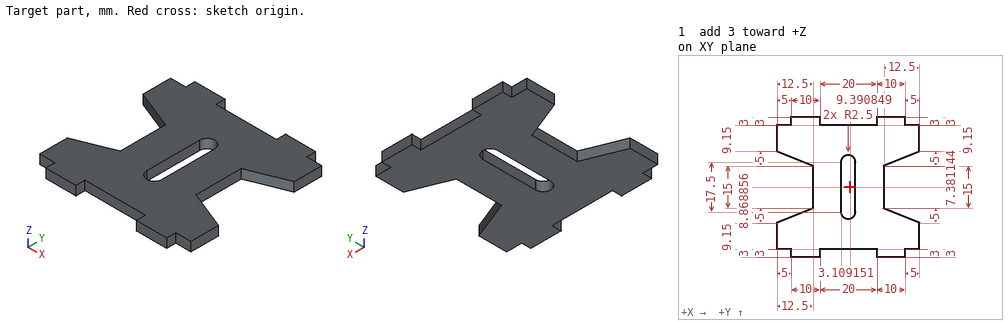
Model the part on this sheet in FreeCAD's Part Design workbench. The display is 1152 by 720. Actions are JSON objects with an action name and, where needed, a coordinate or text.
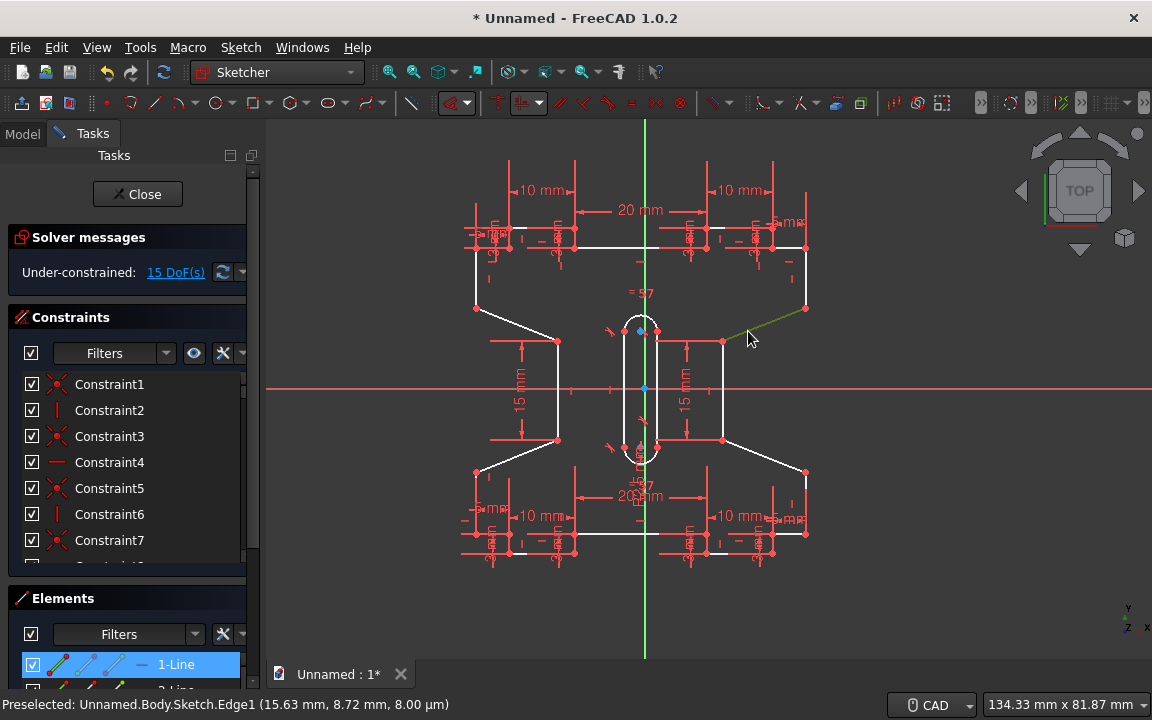
{"action": "left_click", "coordinate": [470, 104]}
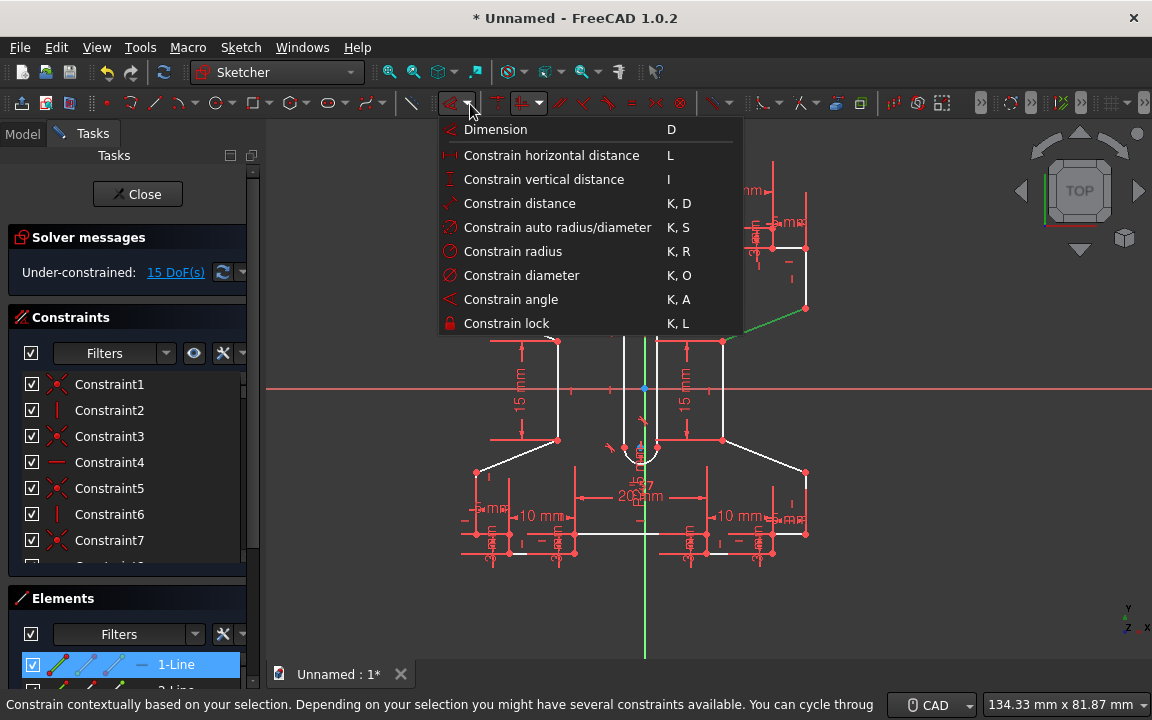
{"action": "left_click", "coordinate": [591, 179]}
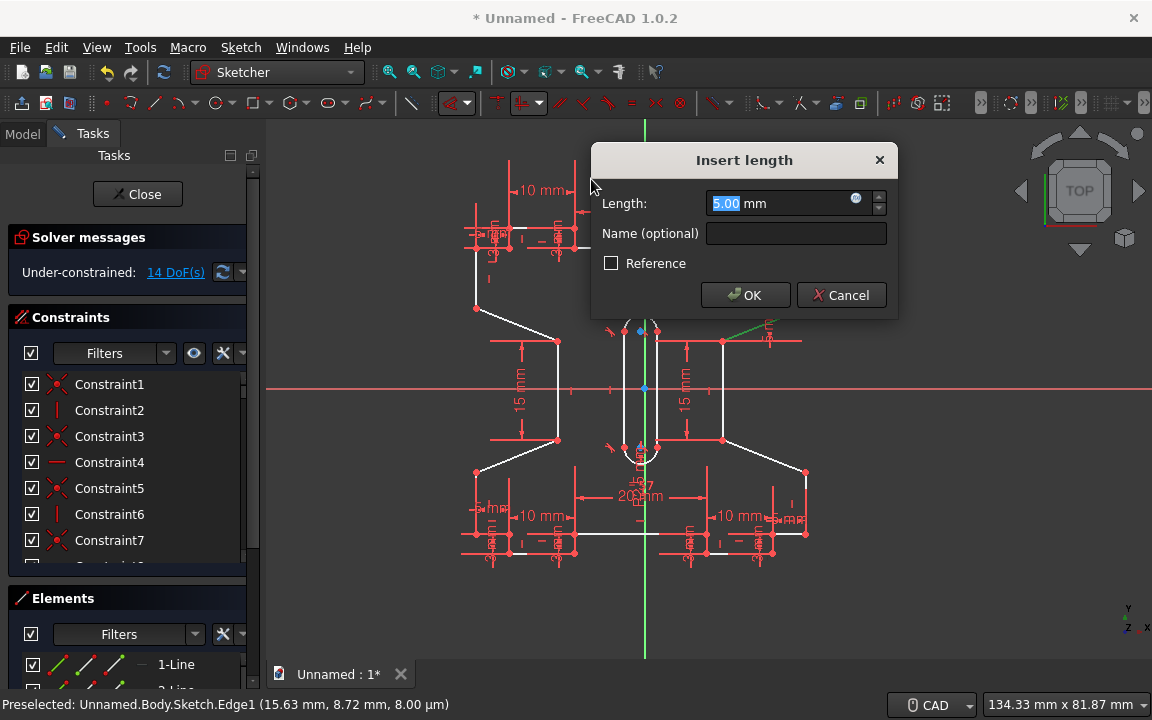
{"action": "type", "text": "5"}
{"action": "key", "text": "Return"}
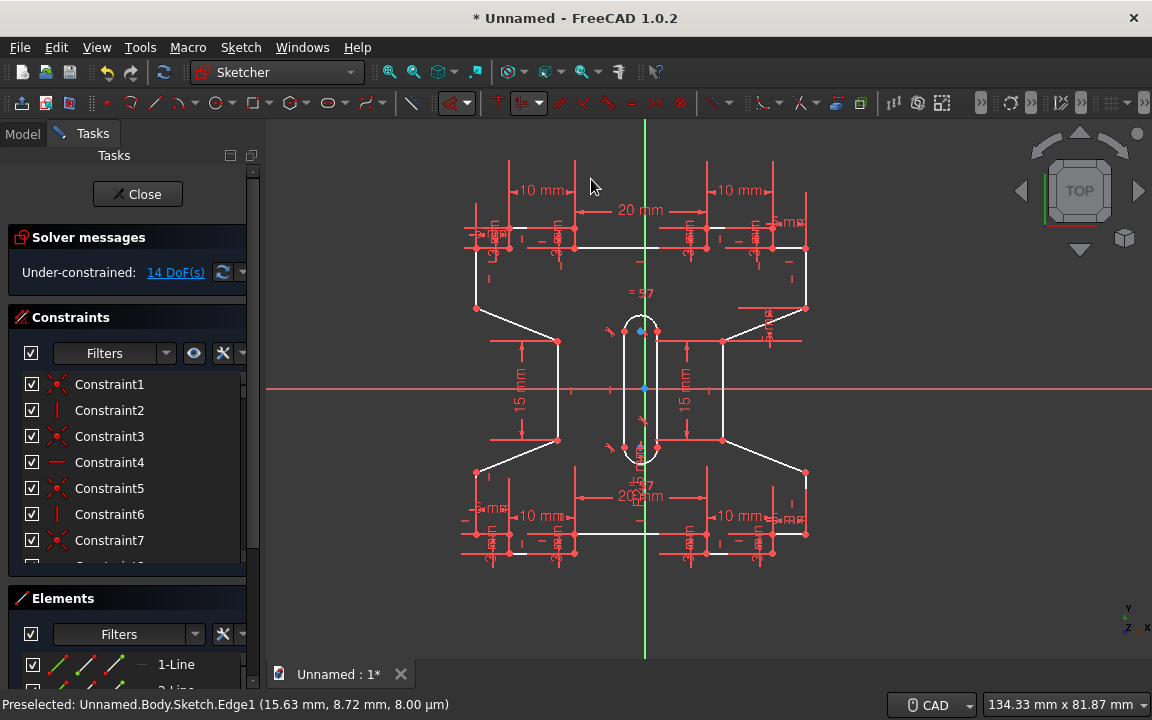
{"action": "left_click", "coordinate": [501, 318]}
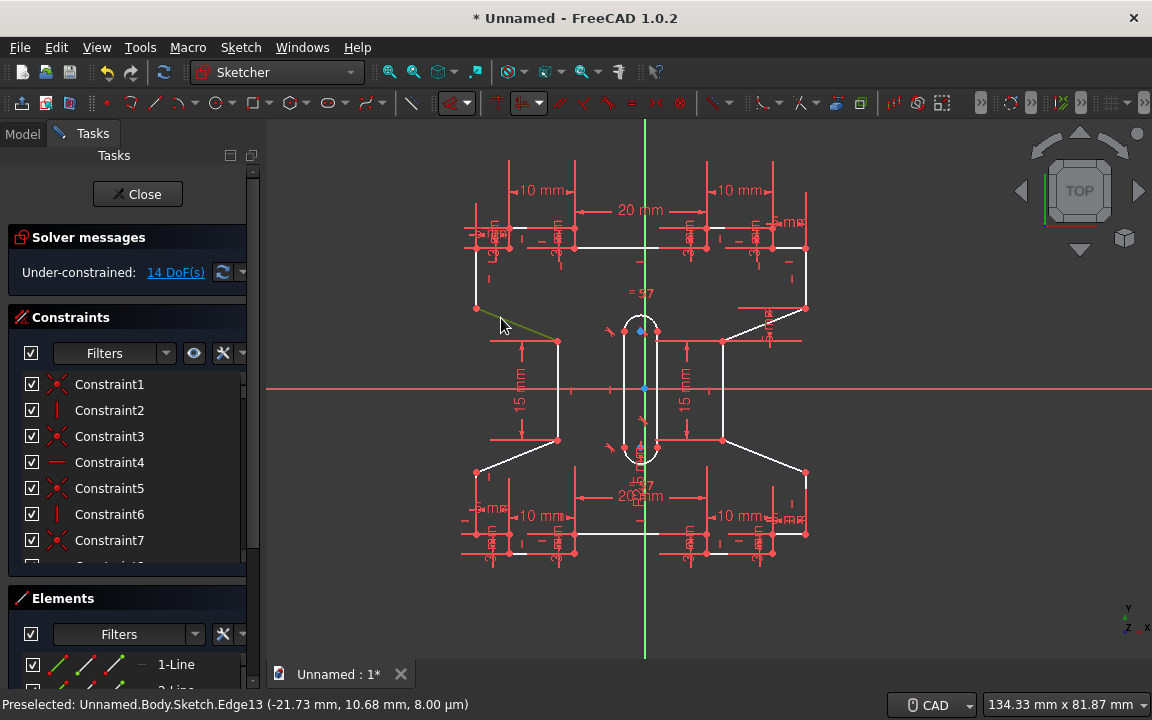
{"action": "left_click", "coordinate": [470, 104]}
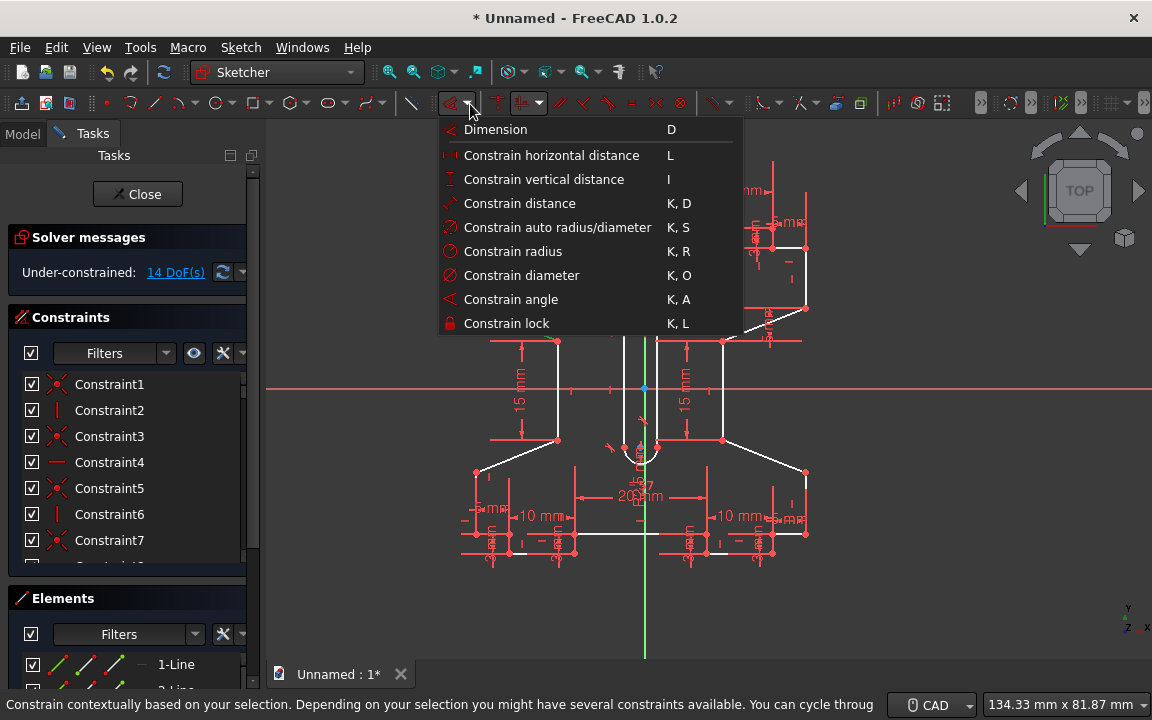
{"action": "left_click", "coordinate": [591, 179]}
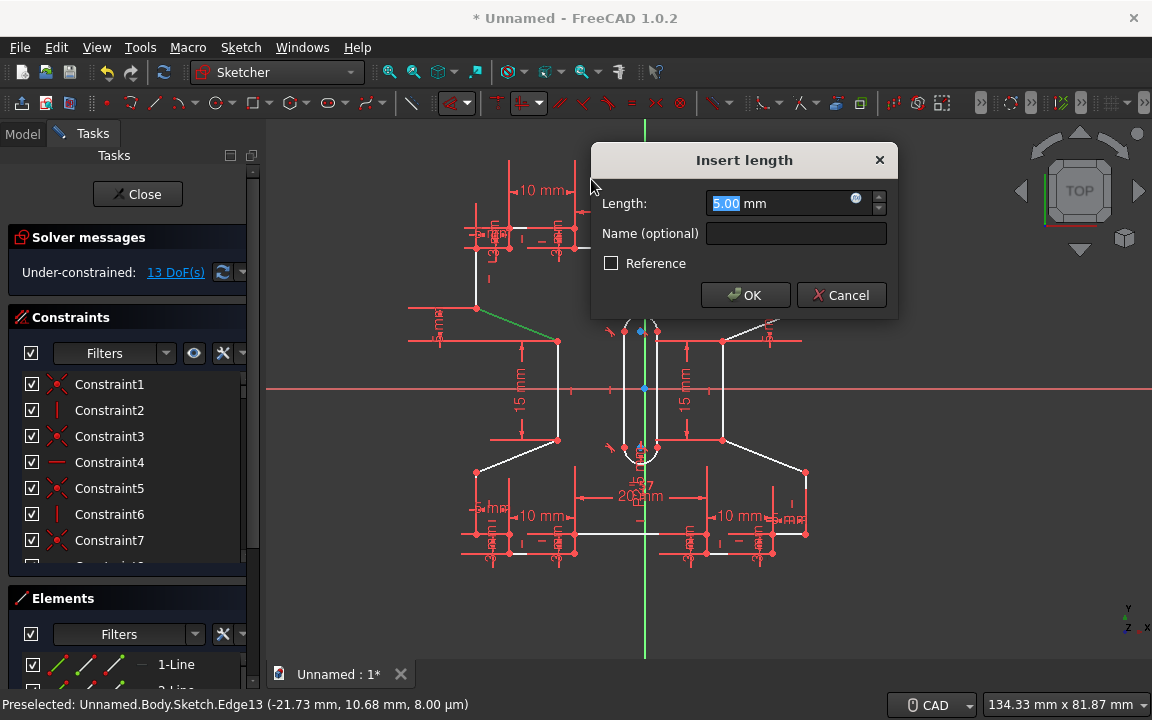
{"action": "type", "text": "5"}
{"action": "key", "text": "Return"}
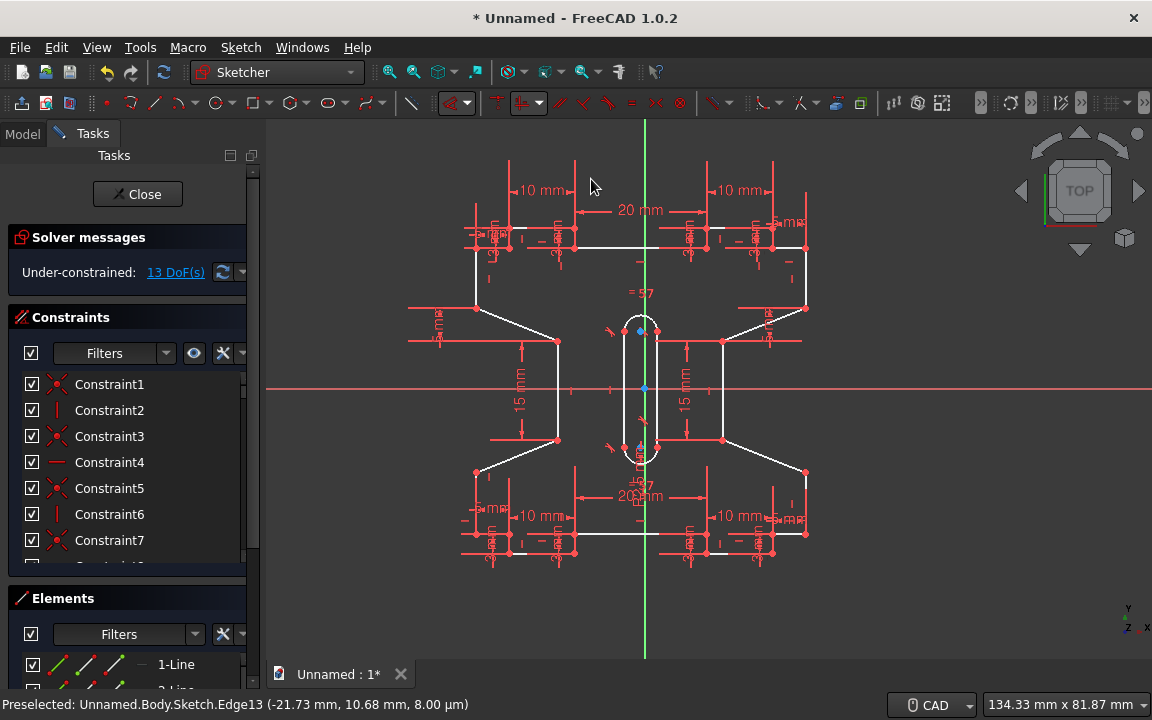
{"action": "left_click", "coordinate": [533, 450]}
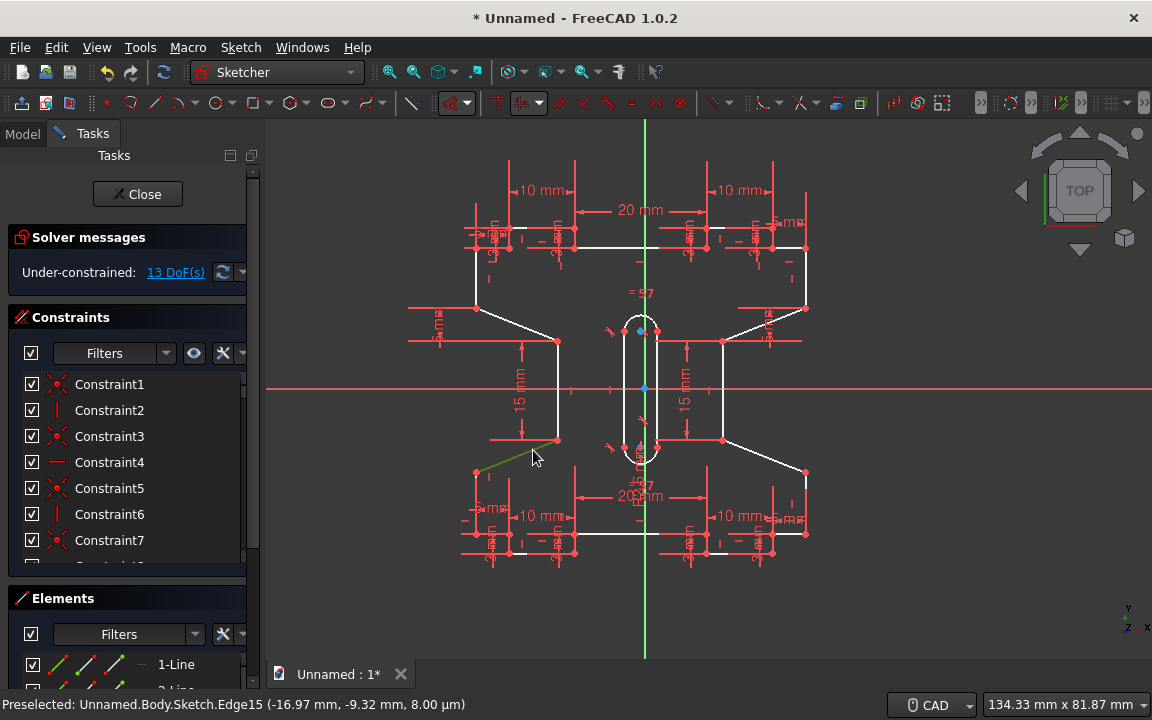
{"action": "key", "text": "i"}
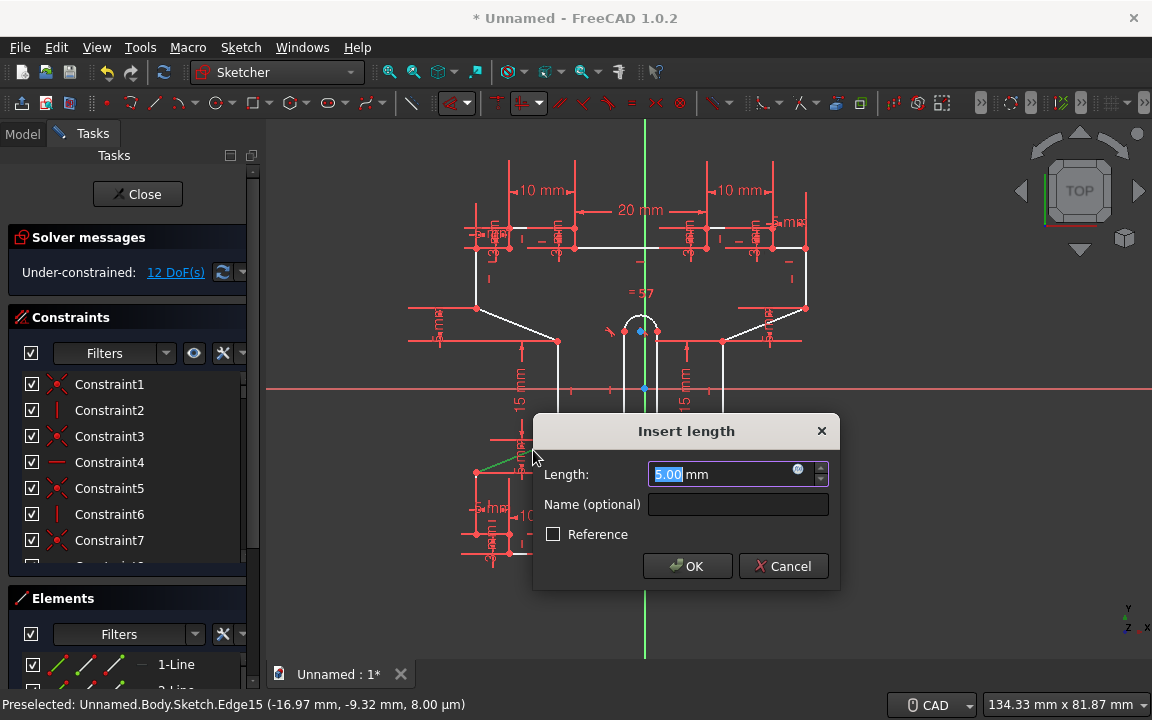
{"action": "type", "text": "5"}
{"action": "key", "text": "Return"}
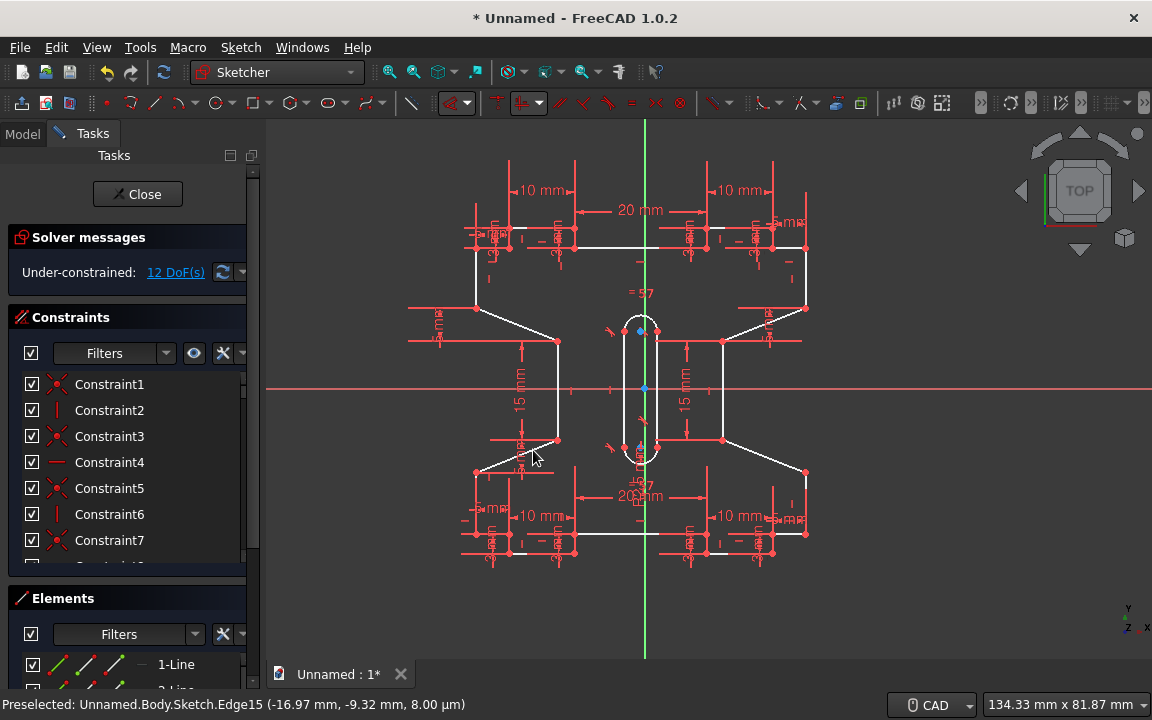
{"action": "left_click", "coordinate": [781, 463]}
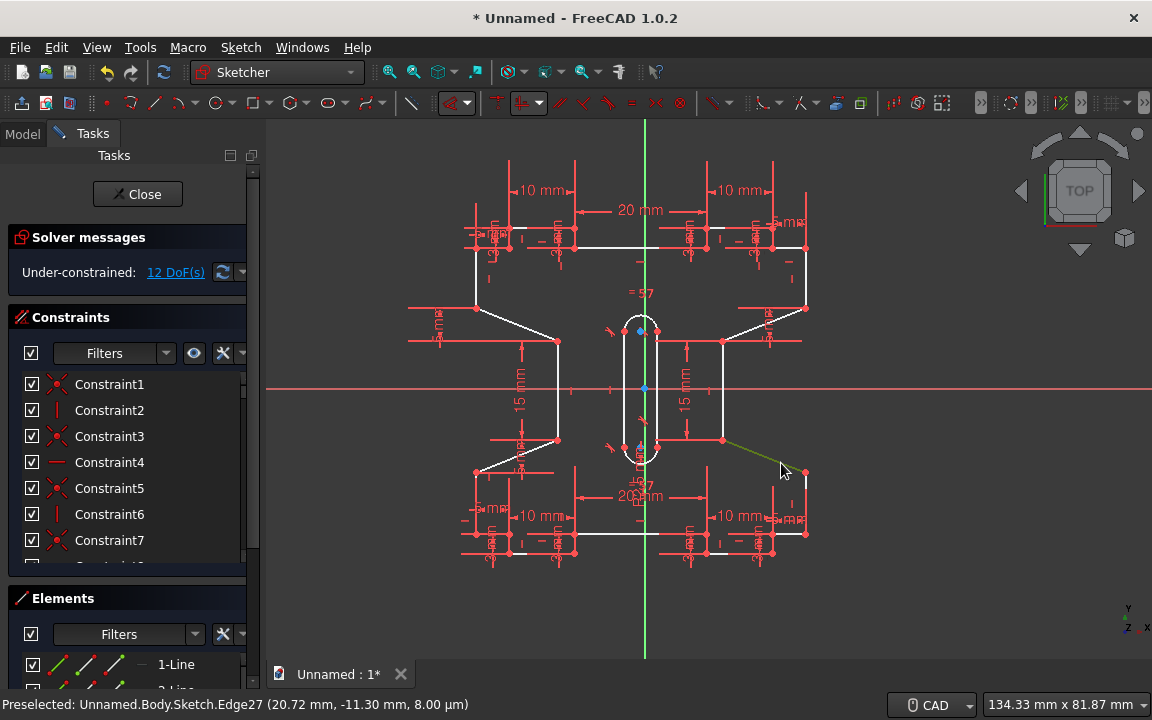
{"action": "left_click", "coordinate": [470, 104]}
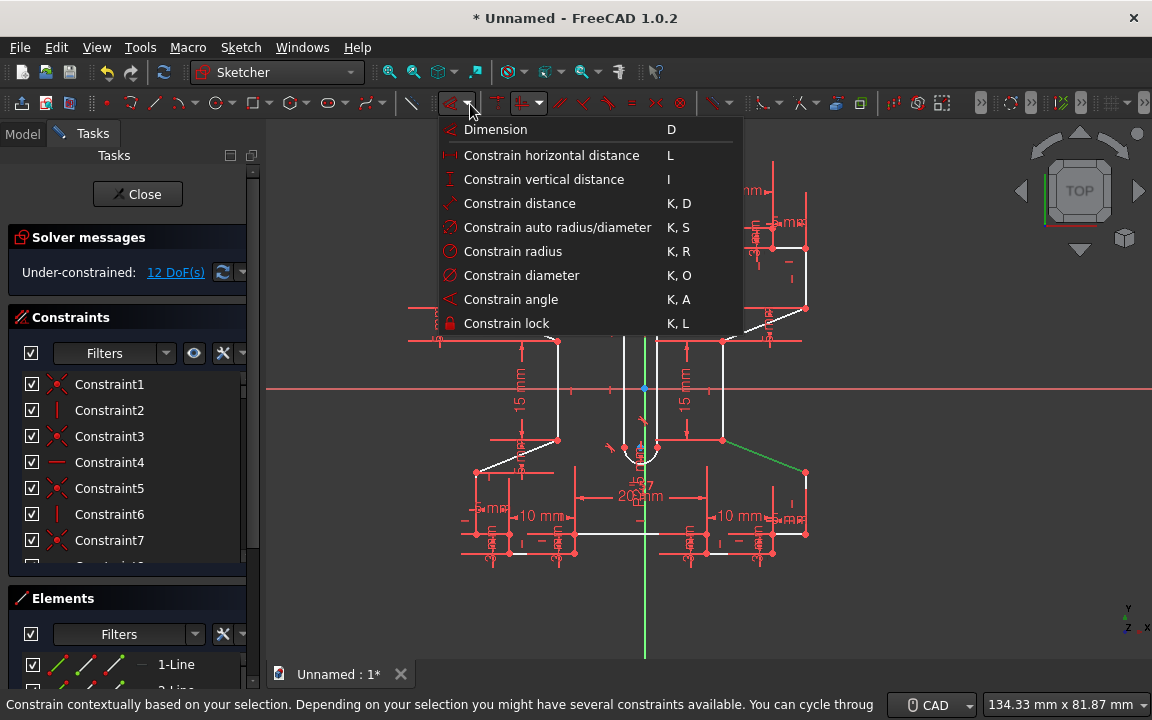
{"action": "left_click", "coordinate": [591, 179]}